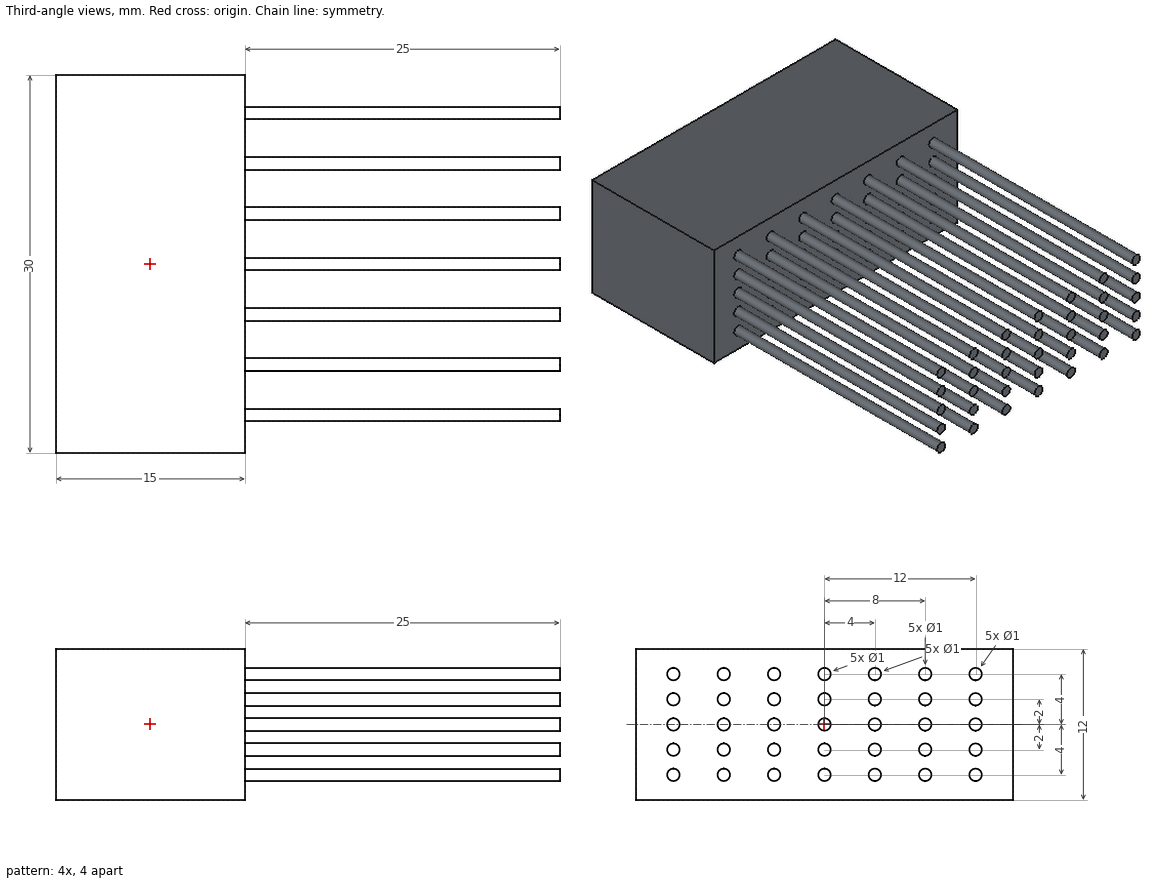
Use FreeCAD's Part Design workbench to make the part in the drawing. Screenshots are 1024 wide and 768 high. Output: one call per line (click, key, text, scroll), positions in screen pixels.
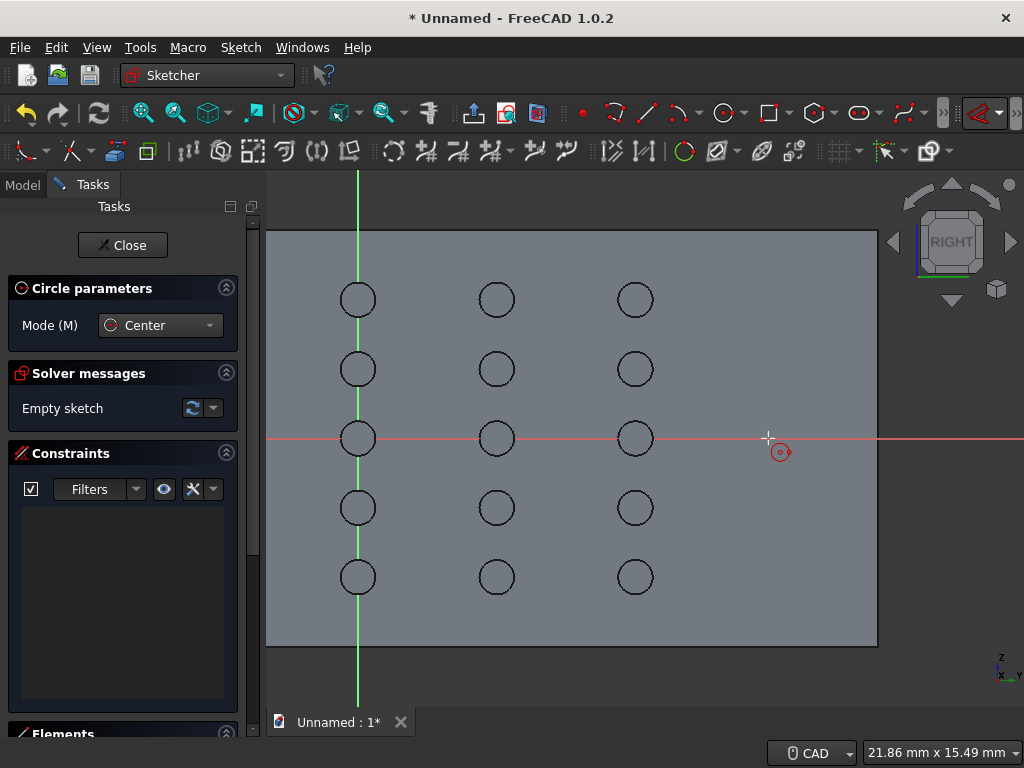
scroll(774, 300, up, 2)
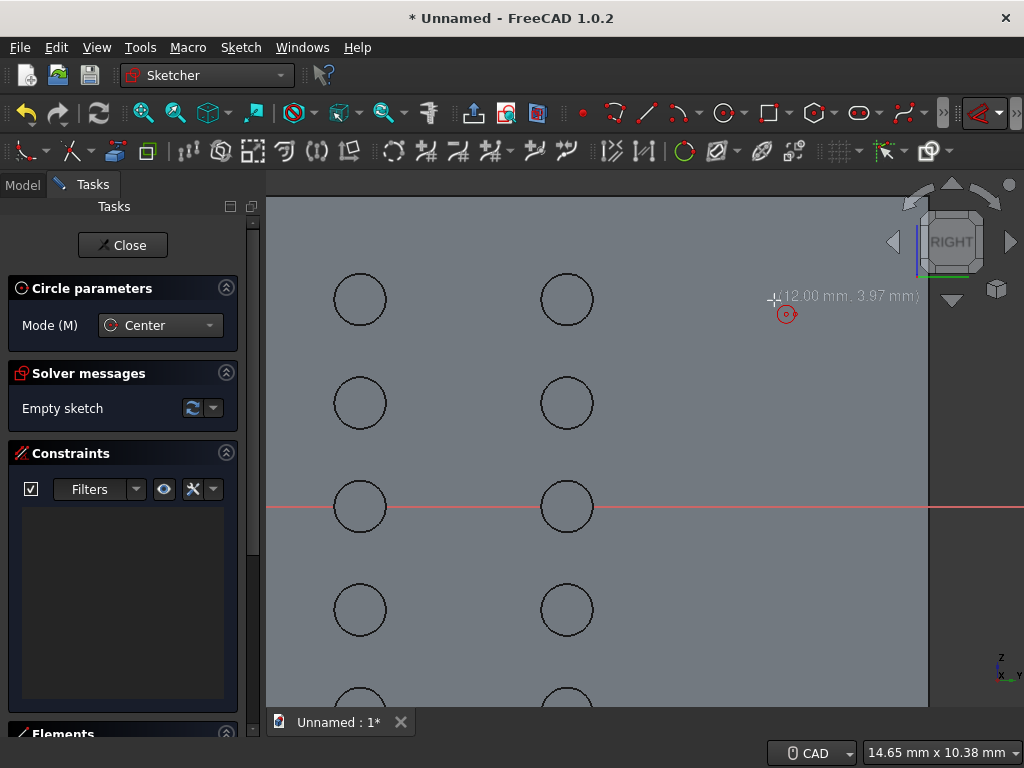
click(774, 300)
move(792, 281)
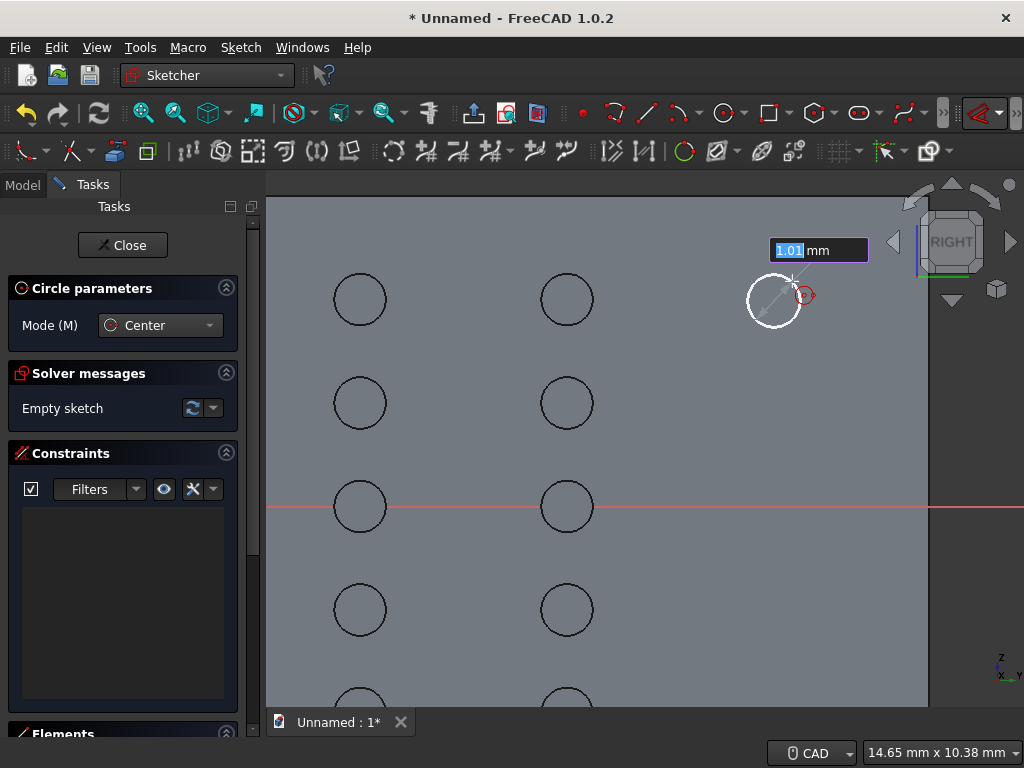
text(1)
key(Return)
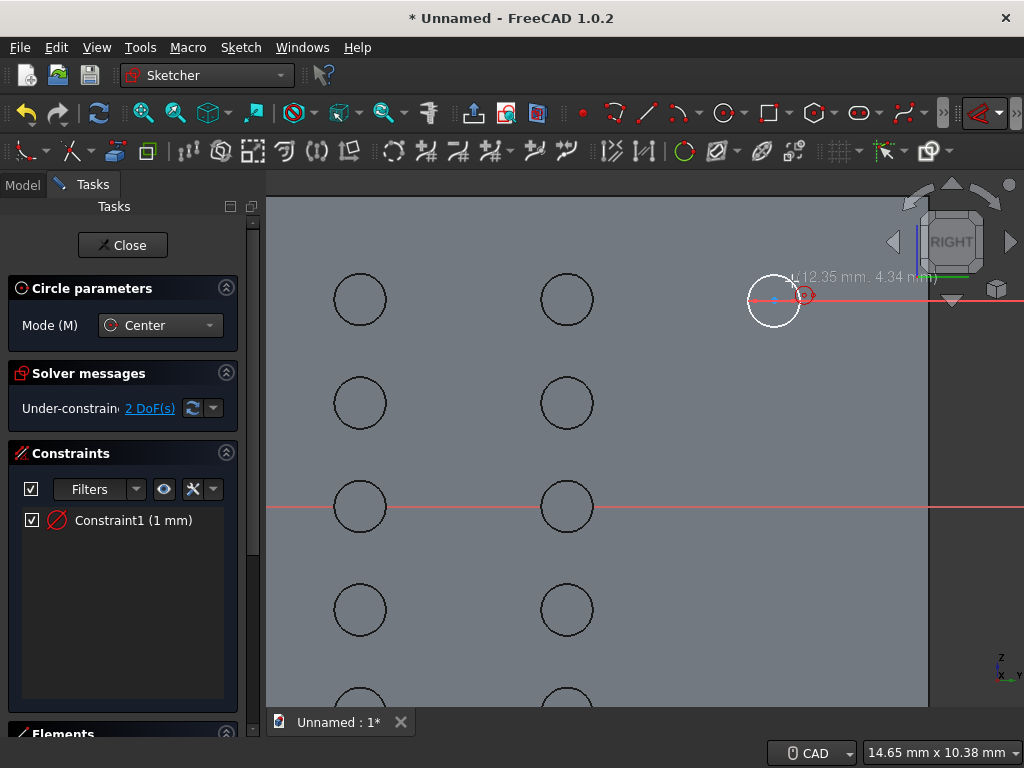
click(774, 403)
move(792, 385)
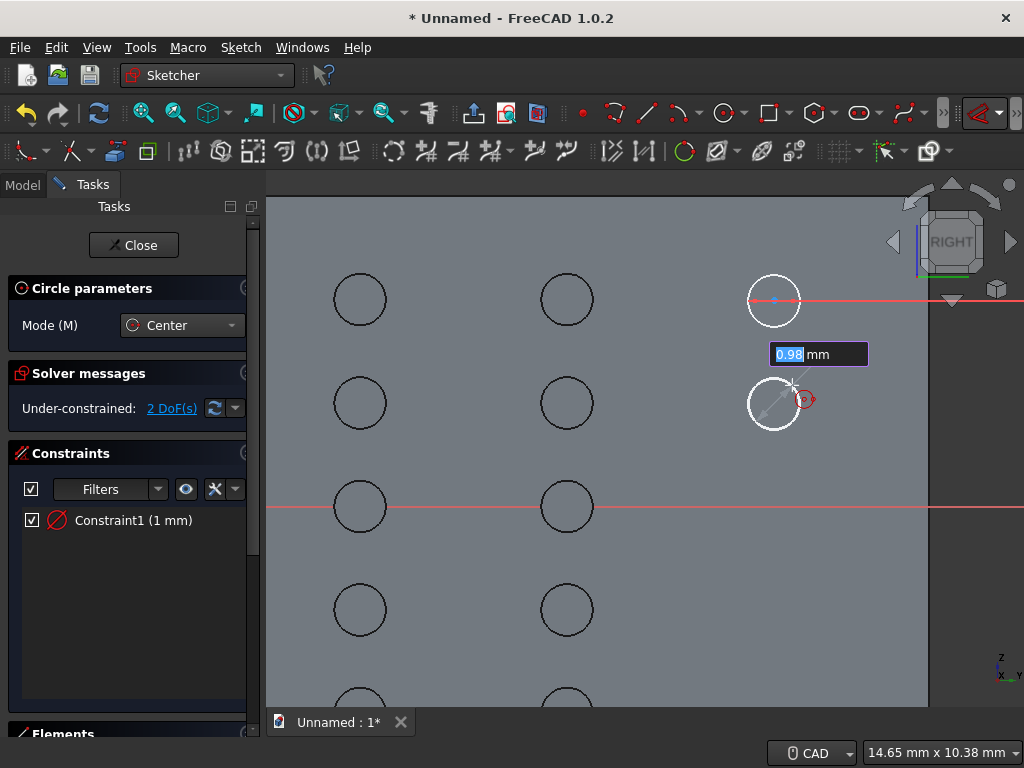
text(1)
key(Return)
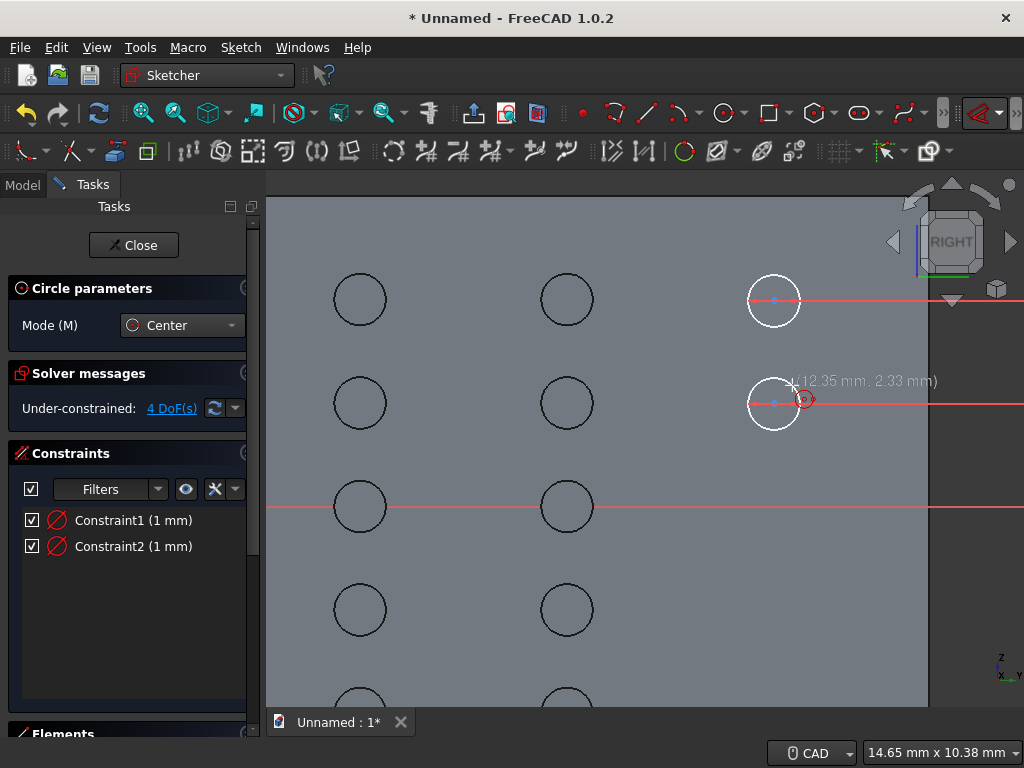
click(774, 506)
move(792, 488)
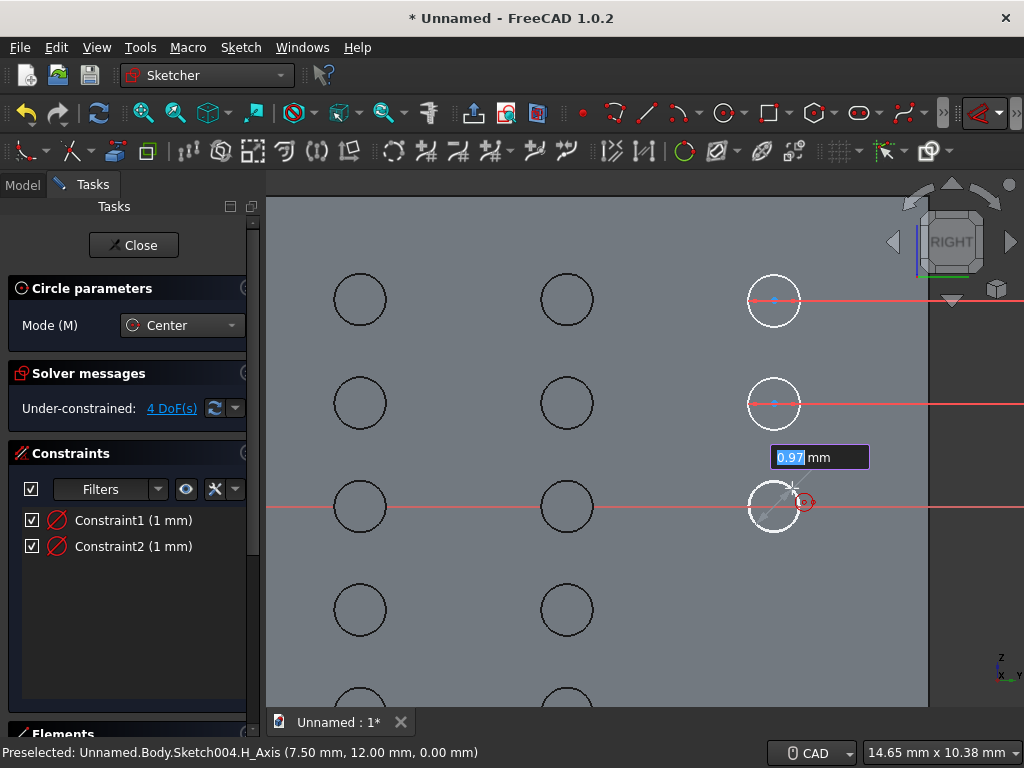
text(1)
key(Return)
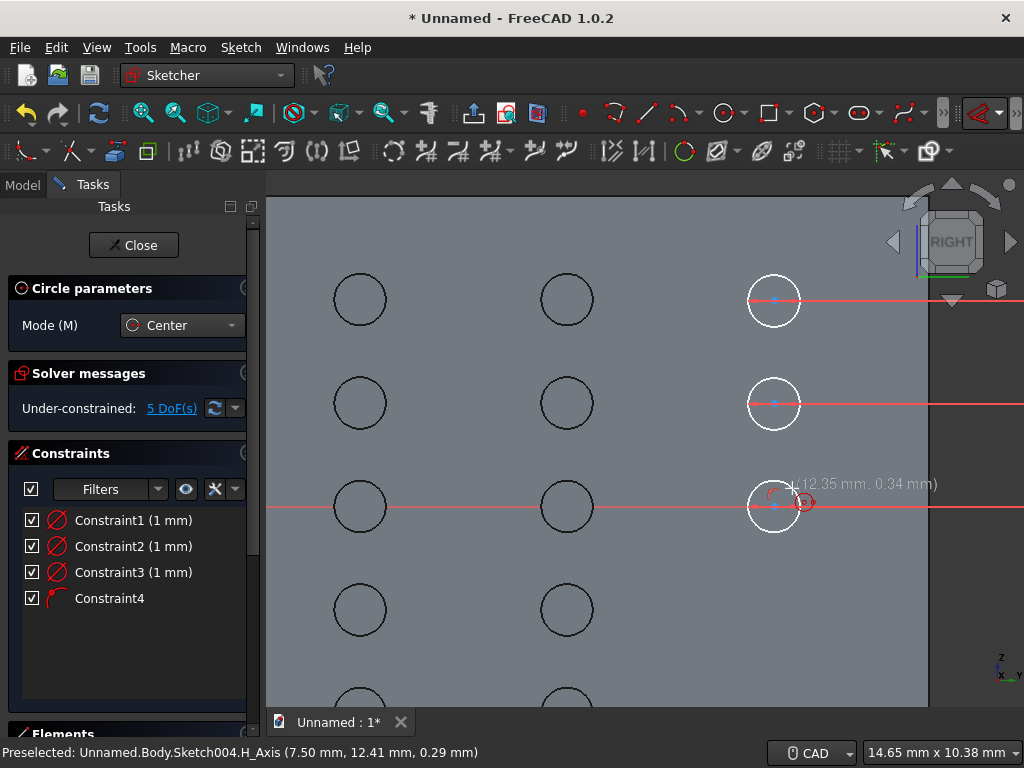
click(774, 610)
move(792, 592)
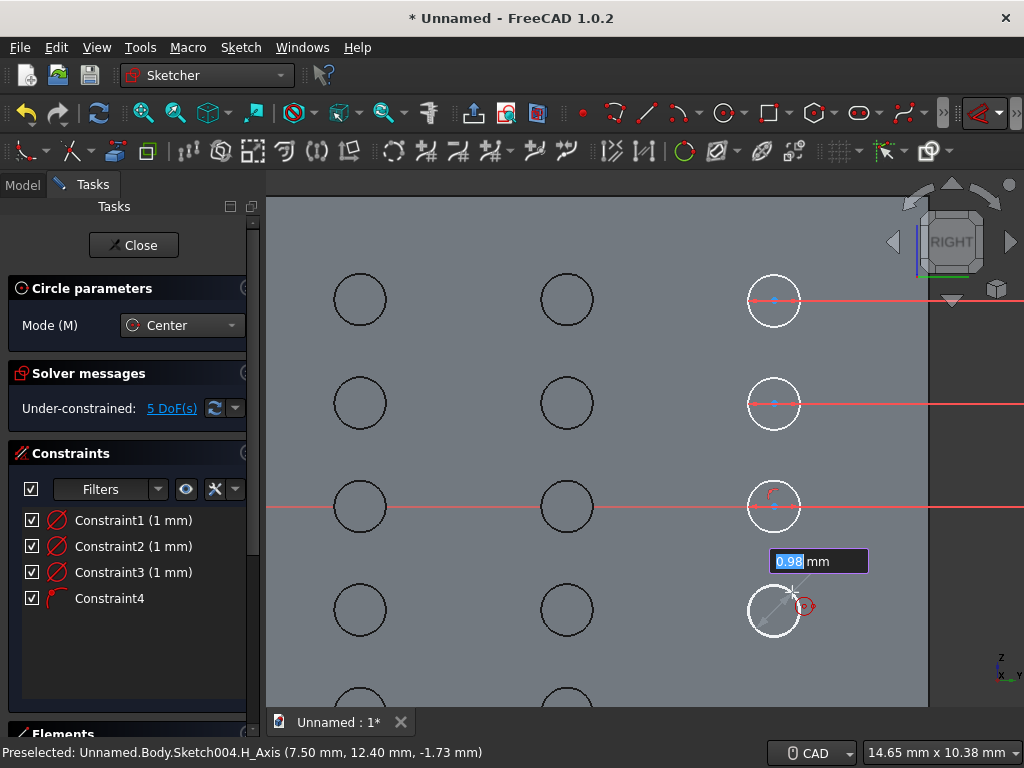
text(1)
key(Return)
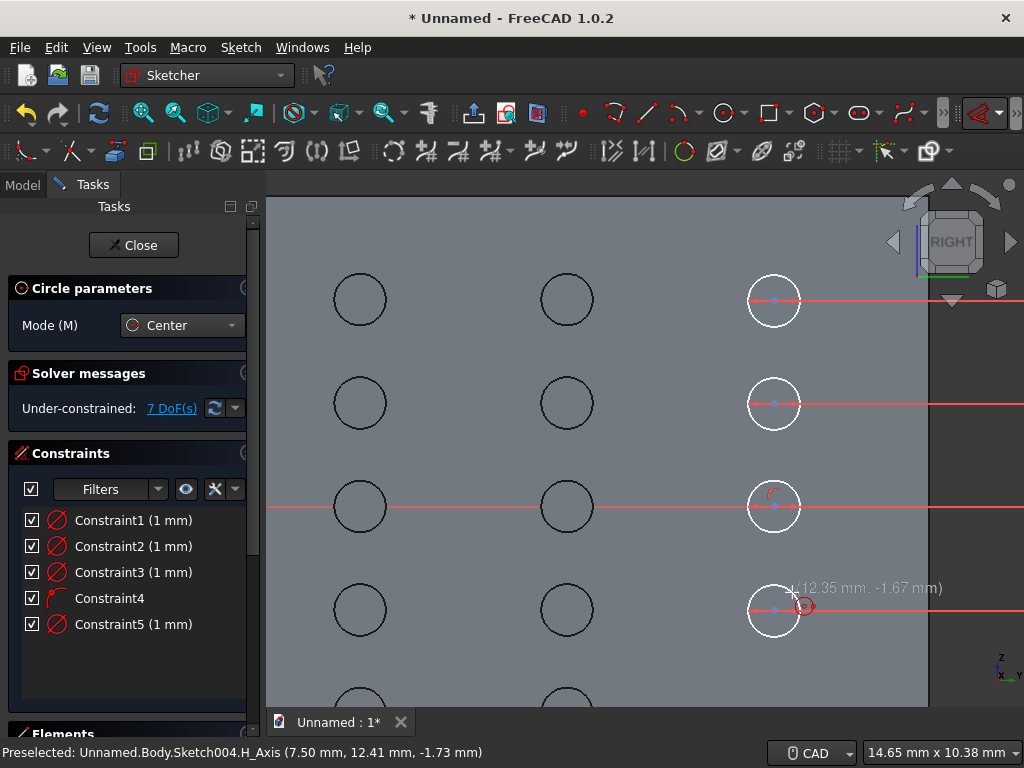
scroll(780, 300, down, 2)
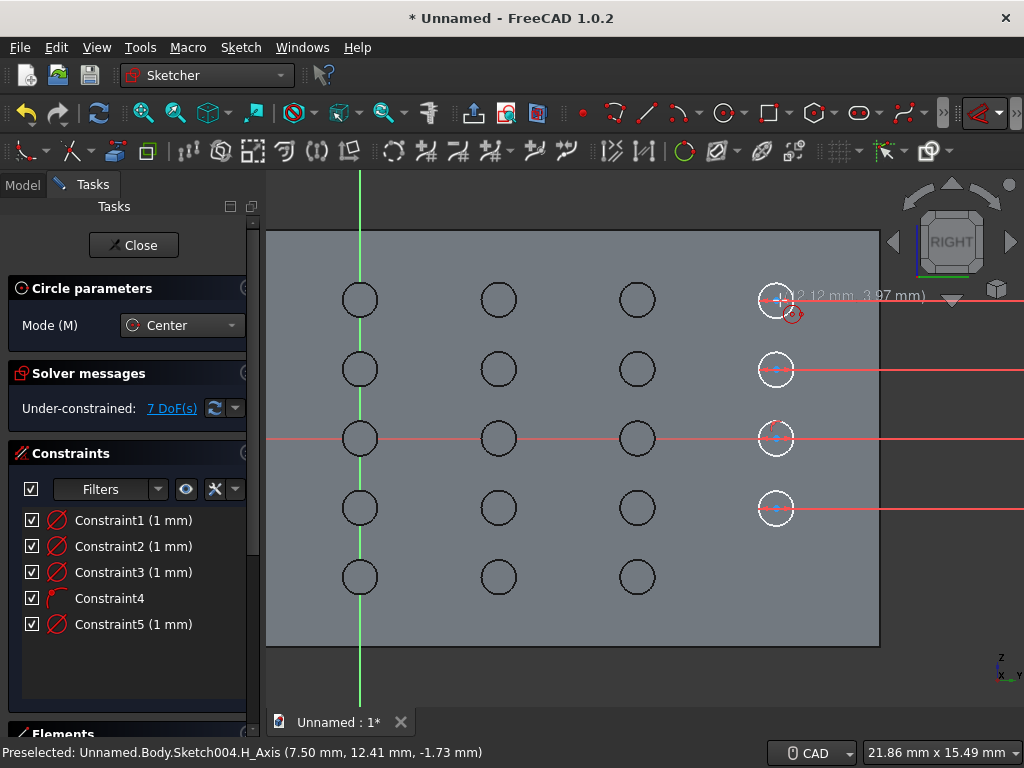
scroll(776, 577, up, 2)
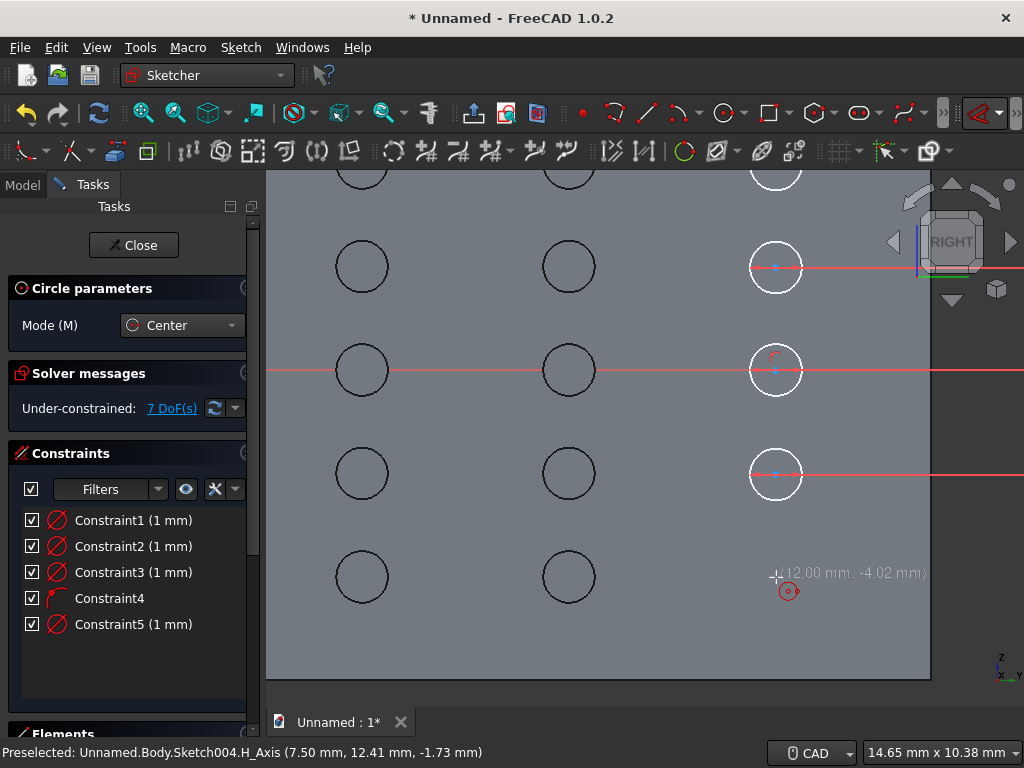
click(776, 577)
move(794, 559)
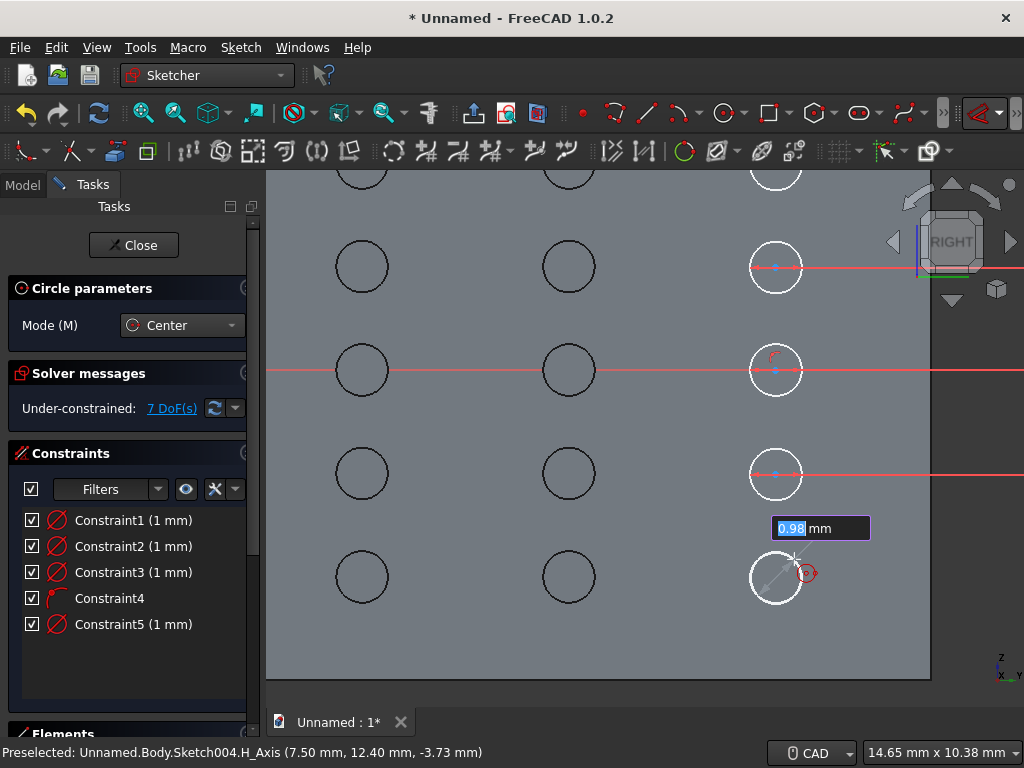
text(1)
key(Return)
key(Escape)